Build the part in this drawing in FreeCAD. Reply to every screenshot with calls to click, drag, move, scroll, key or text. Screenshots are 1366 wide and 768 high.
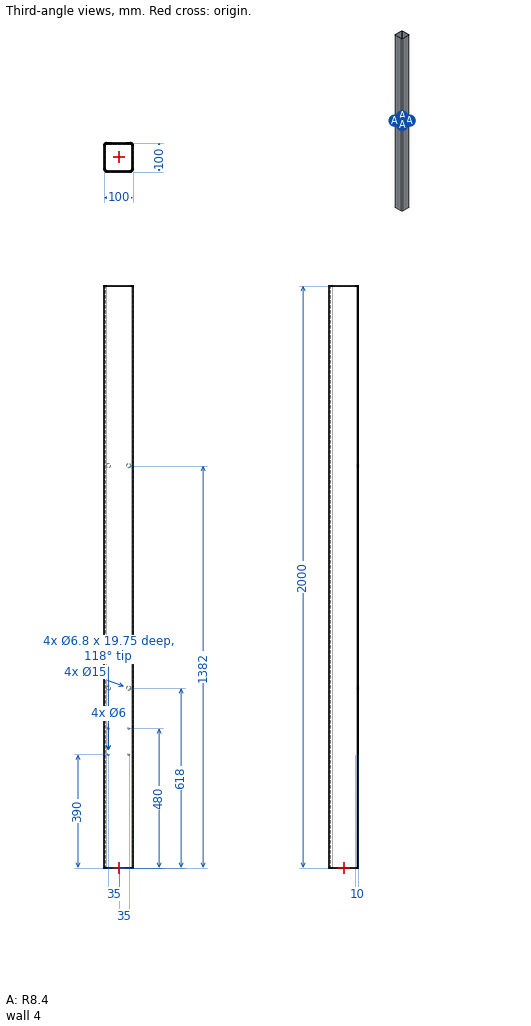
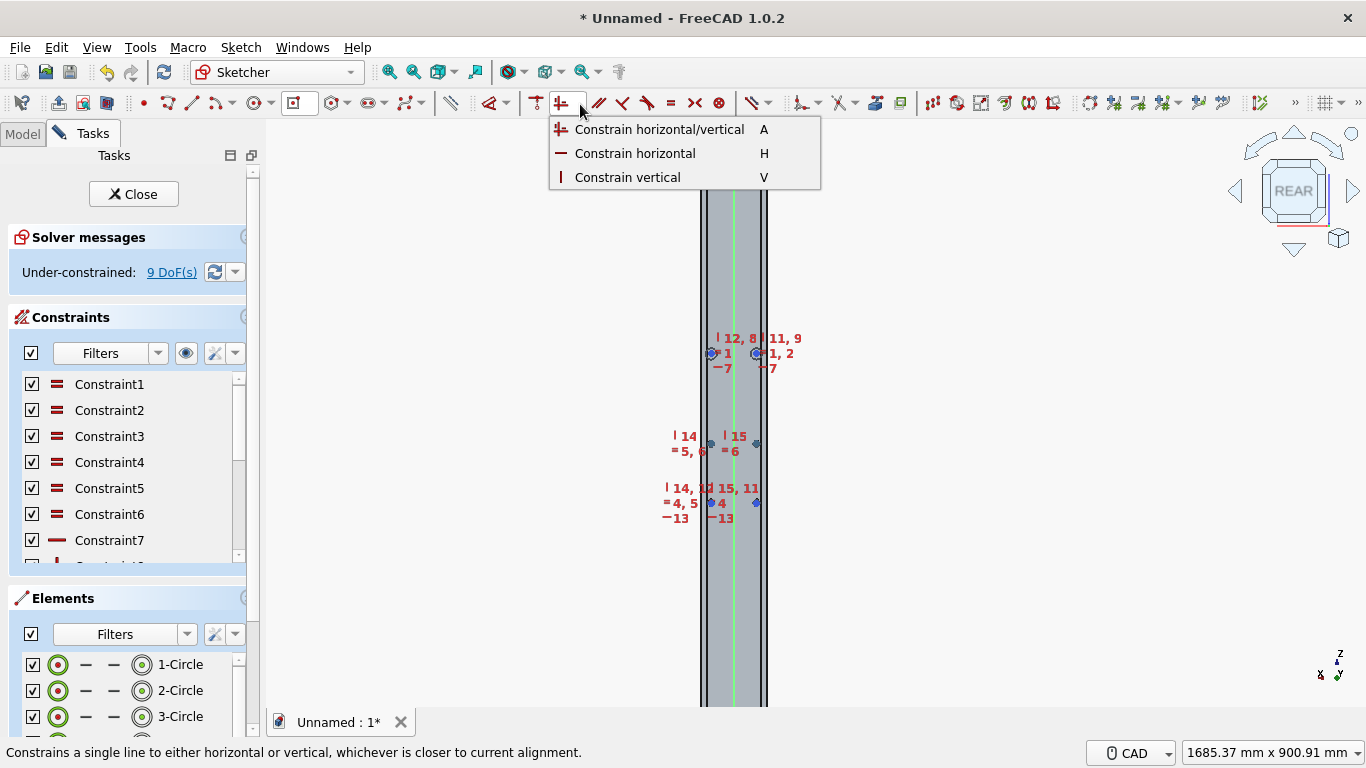
click(685, 153)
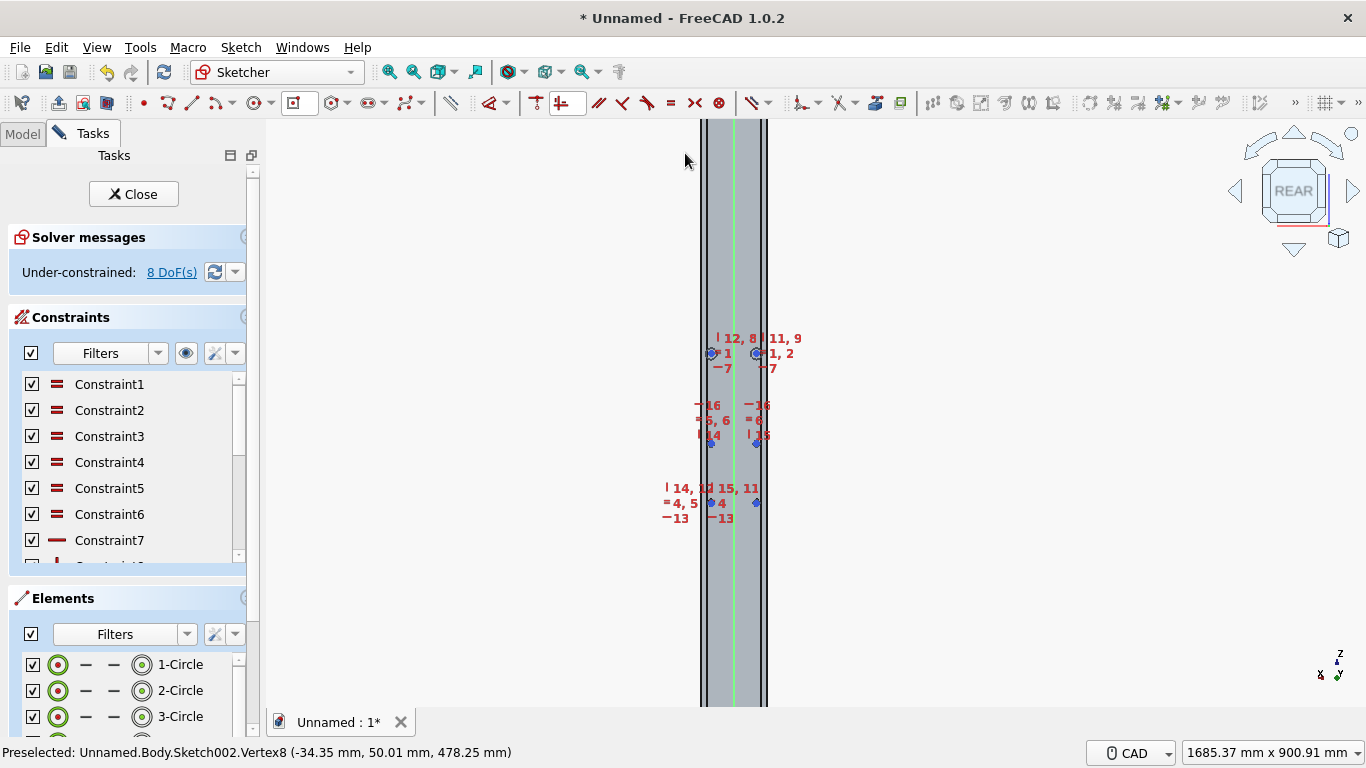
click(490, 104)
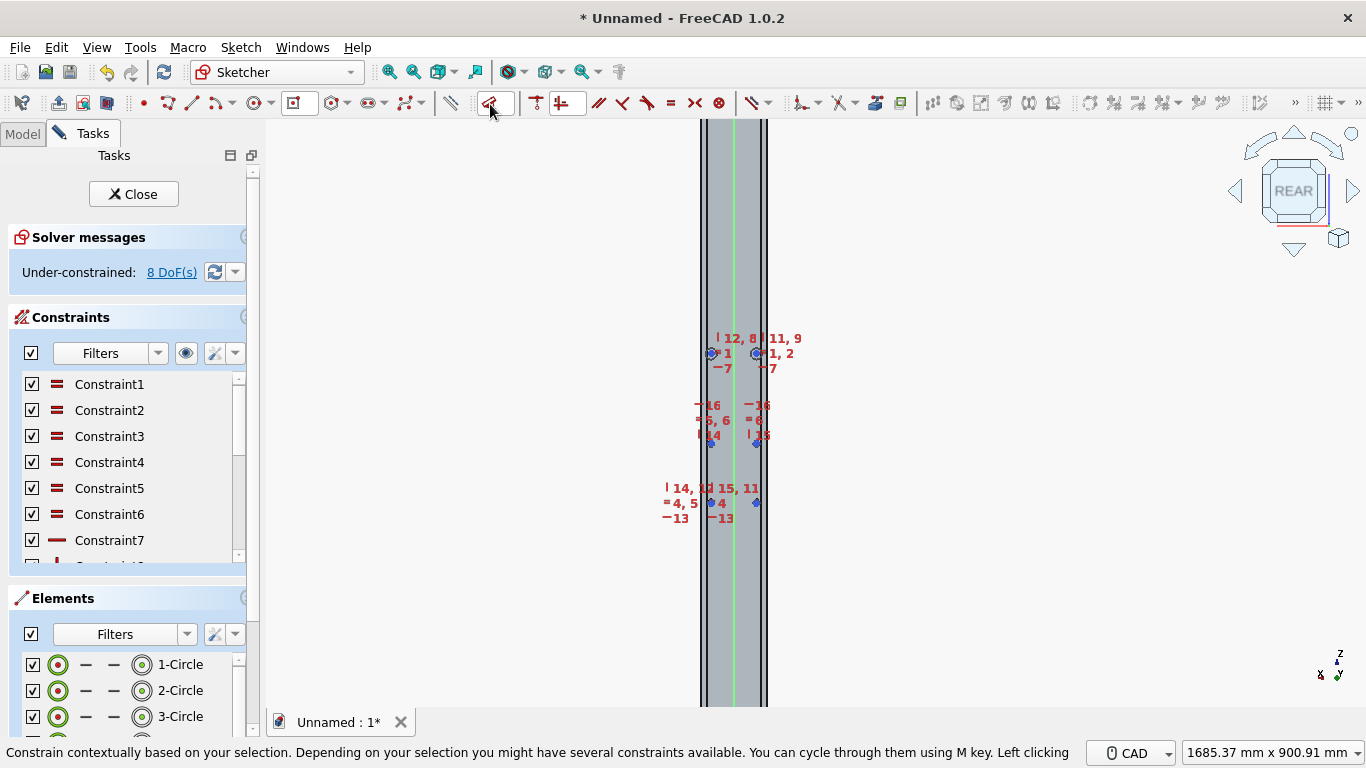
scroll(707, 350, up, 7)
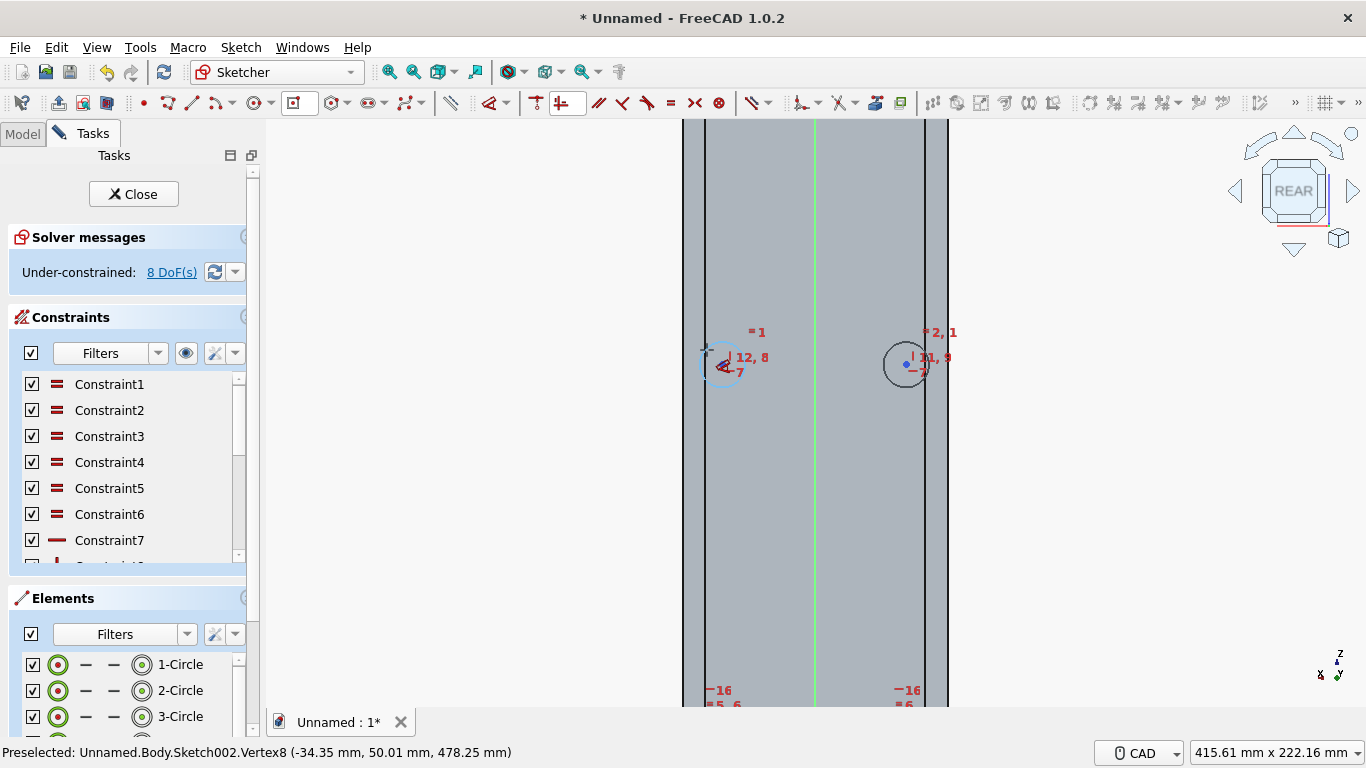
click(706, 349)
click(683, 327)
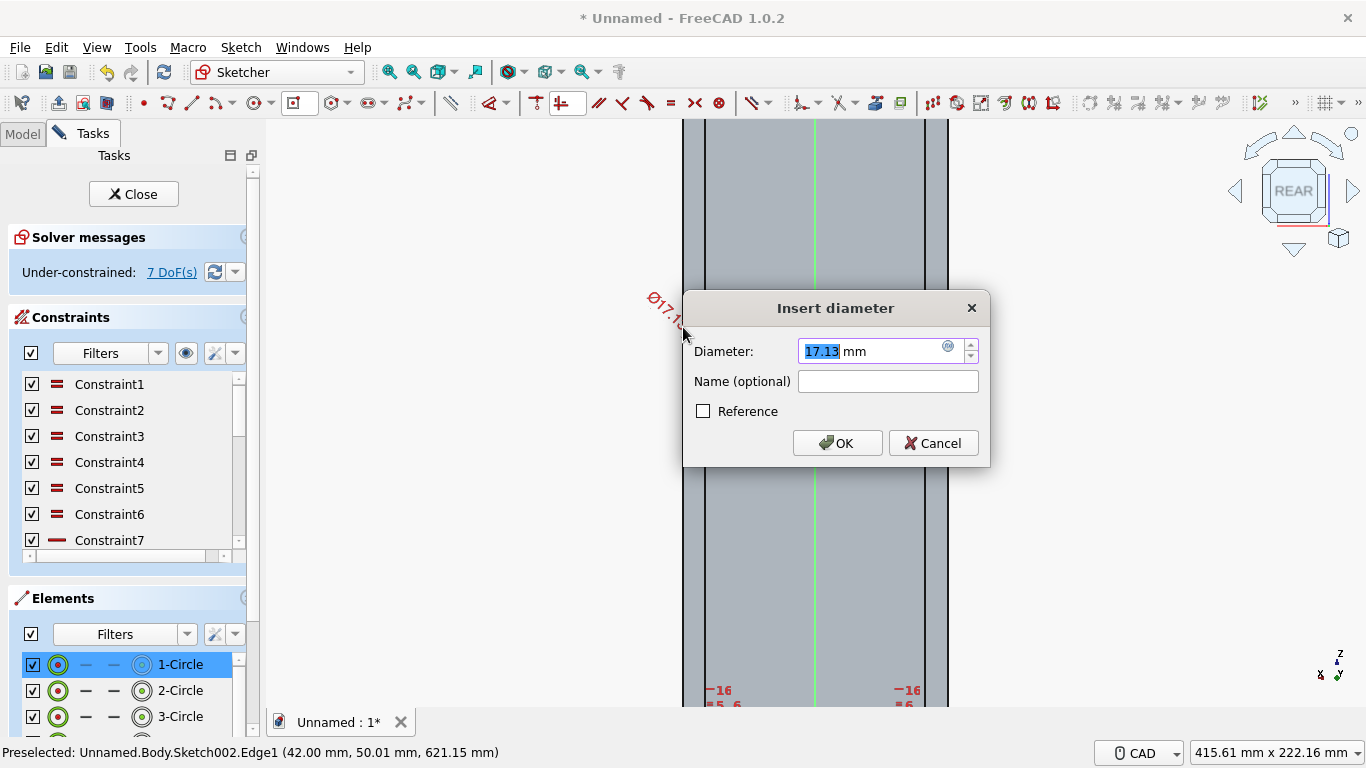
text(15)
key(Return)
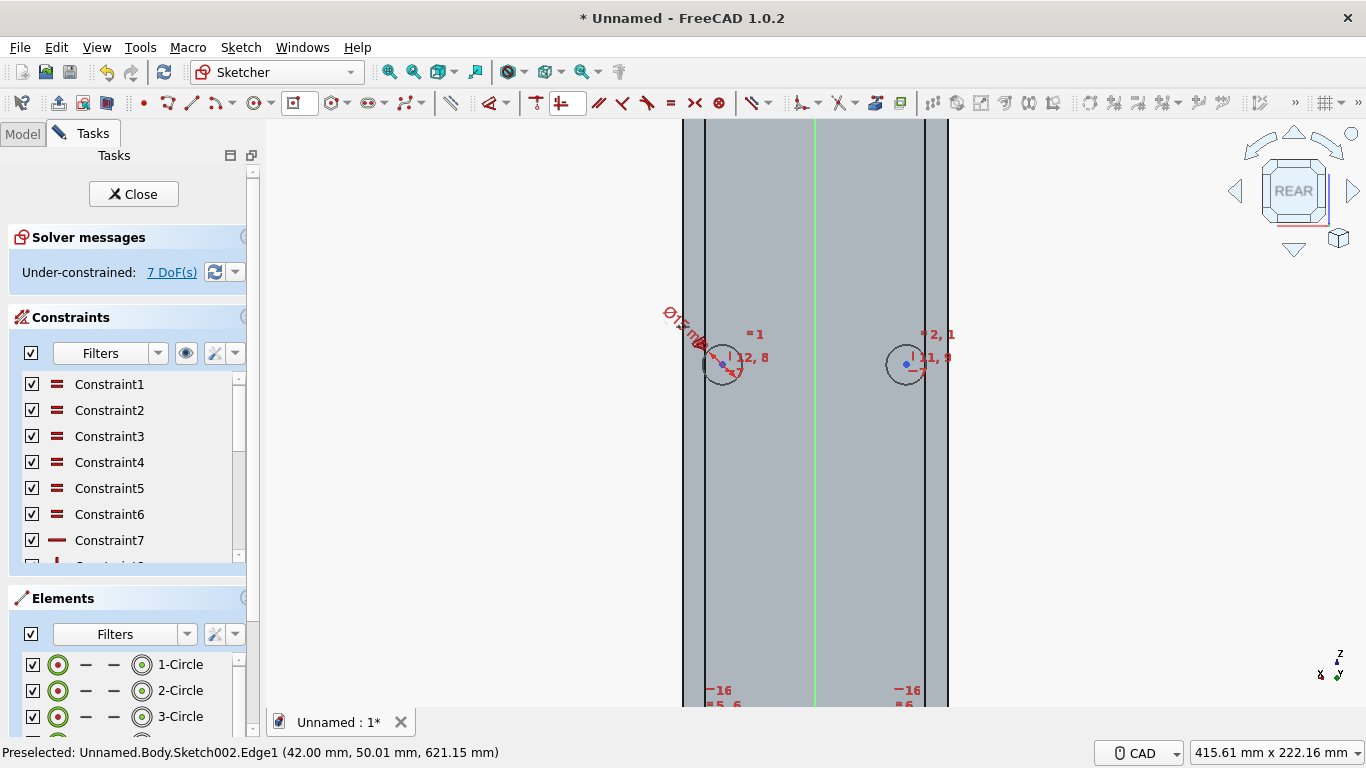
scroll(739, 445, down, 11)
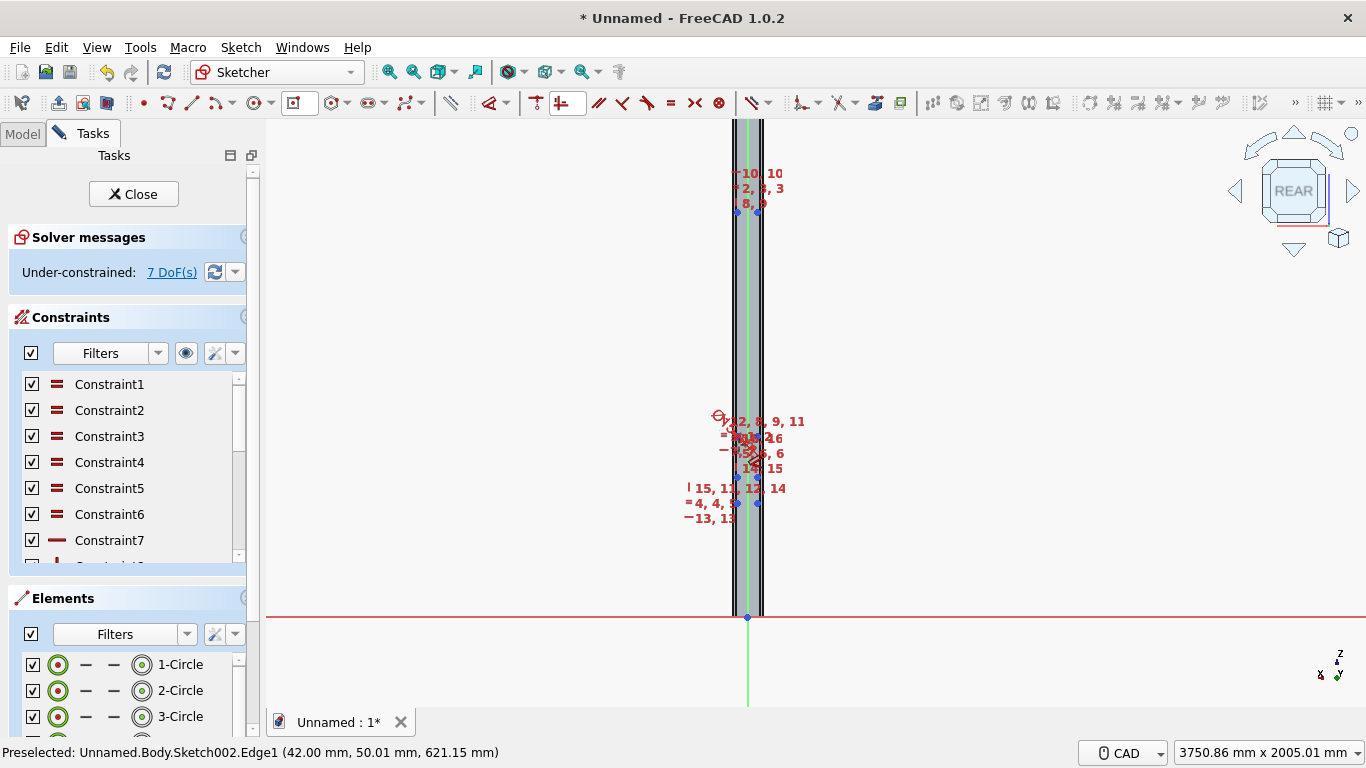
scroll(759, 503, up, 16)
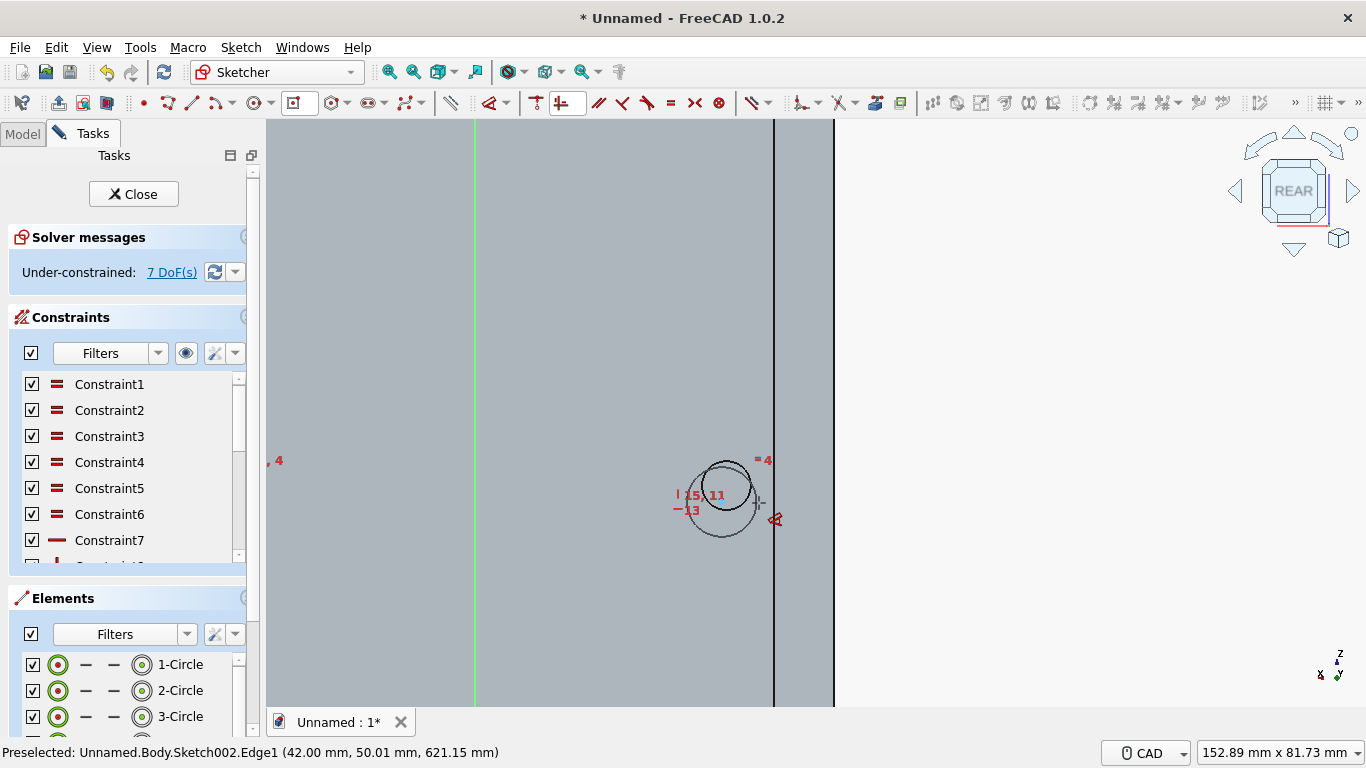
click(746, 477)
click(768, 454)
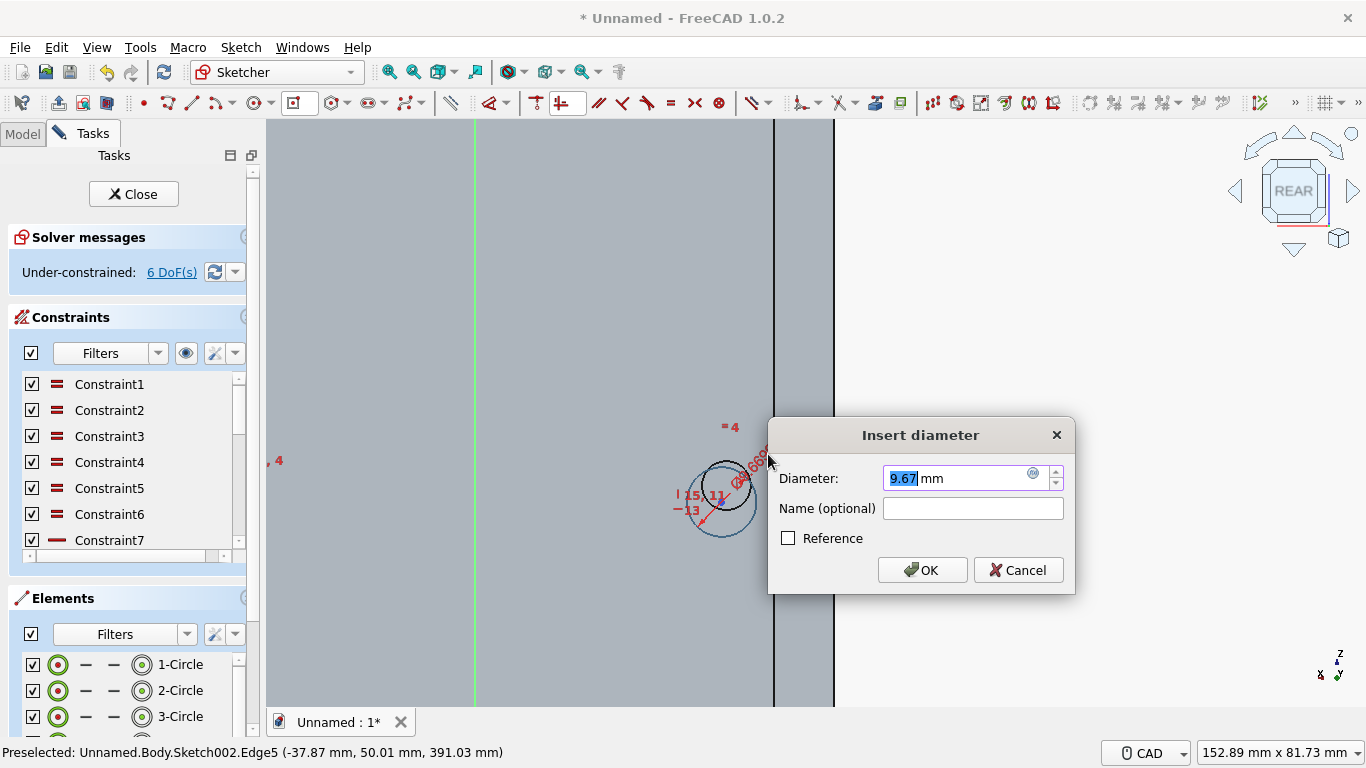
text(6)
key(Return)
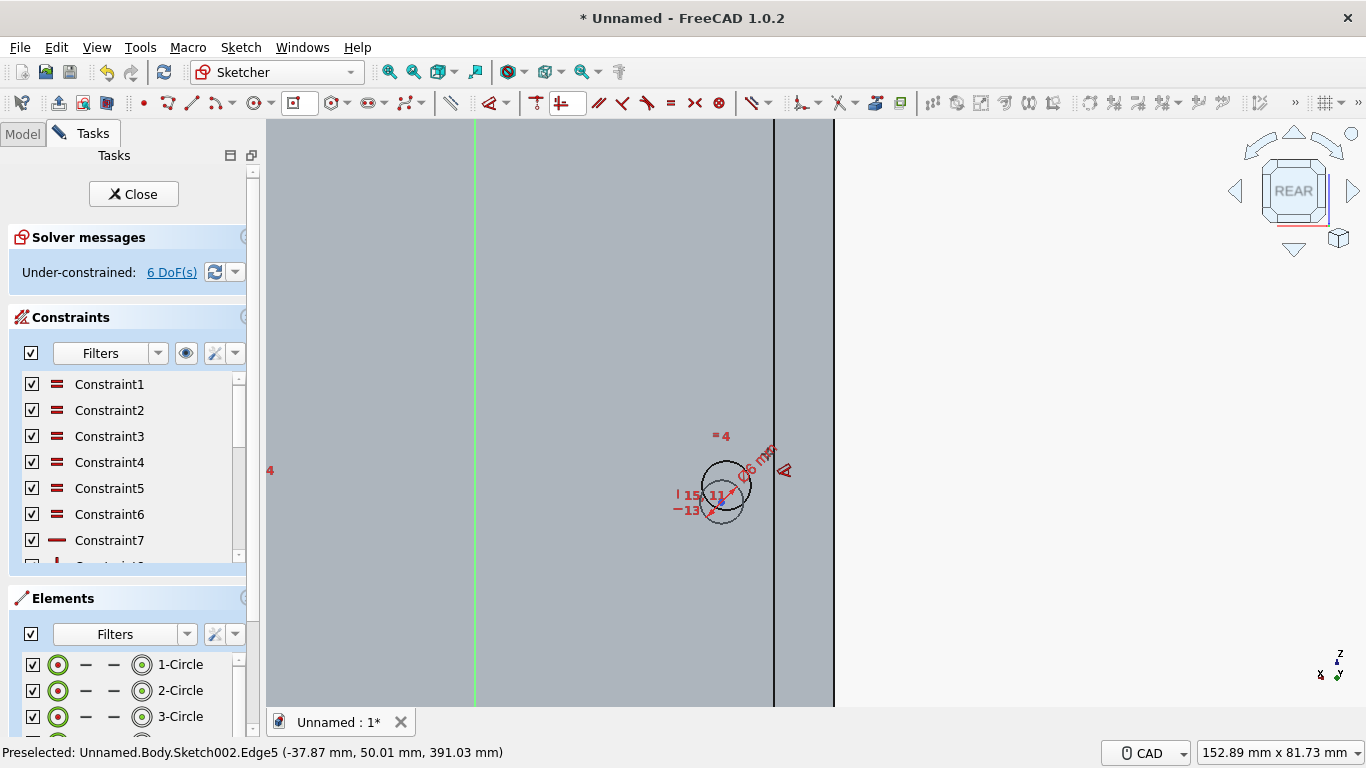
scroll(759, 503, down, 16)